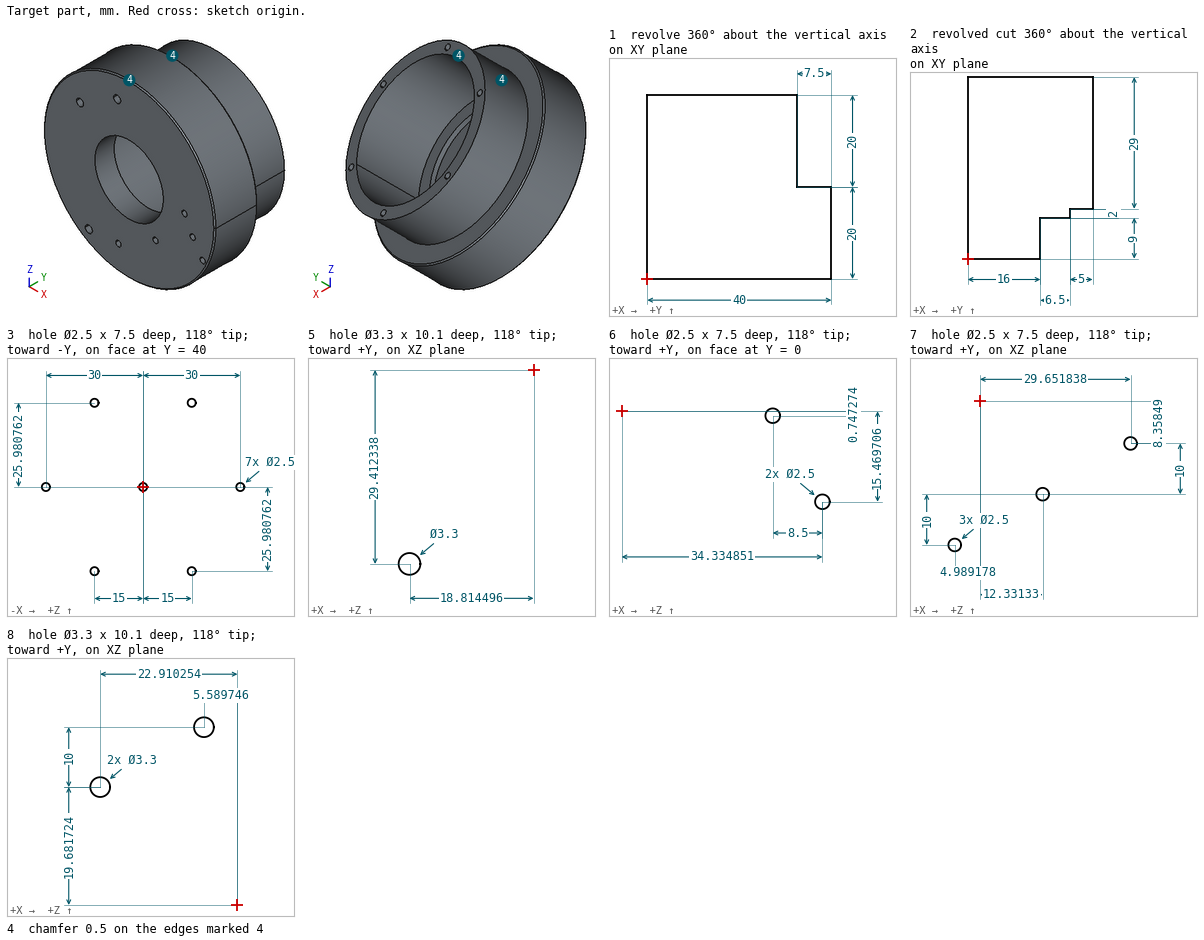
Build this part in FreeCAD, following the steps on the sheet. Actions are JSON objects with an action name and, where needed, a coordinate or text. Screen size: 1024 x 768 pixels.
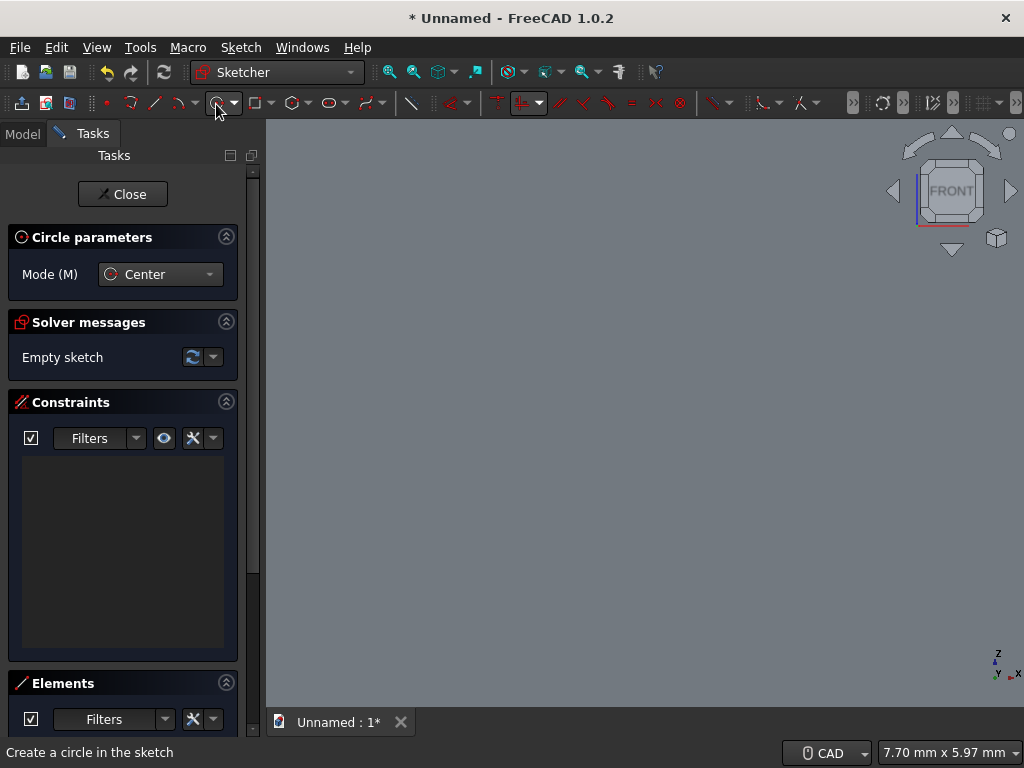
{"action": "left_click", "coordinate": [576, 394]}
{"action": "mouse_move", "coordinate": [691, 279]}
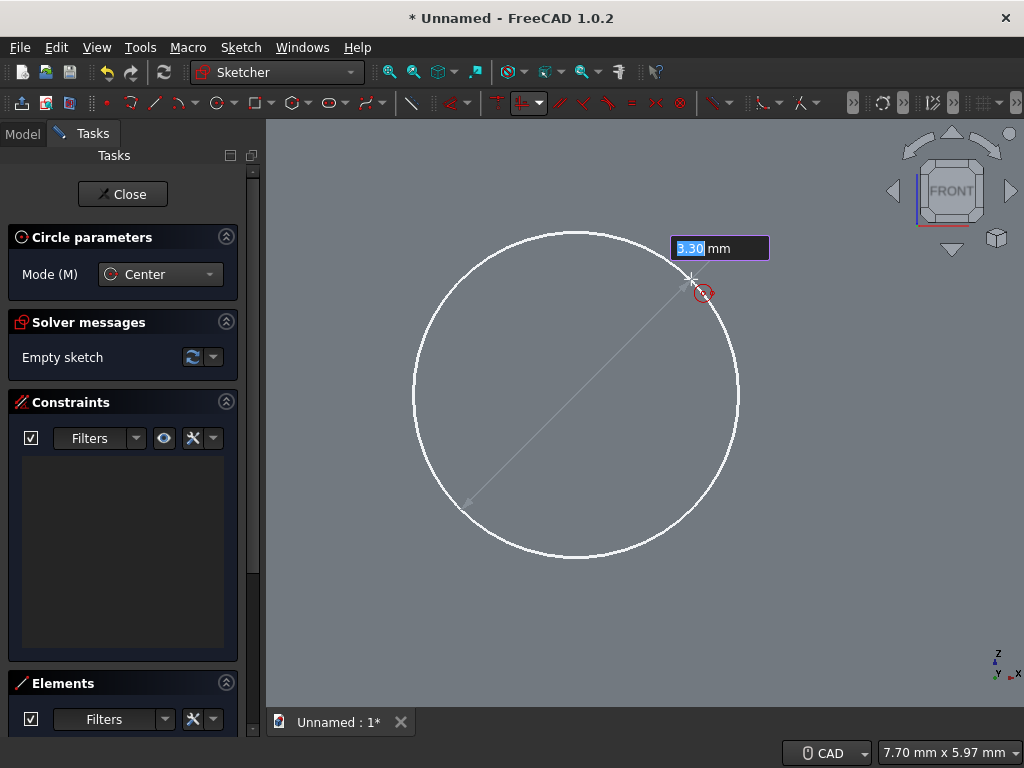
{"action": "type", "text": "3.3"}
{"action": "key", "text": "Return"}
{"action": "key", "text": "Escape"}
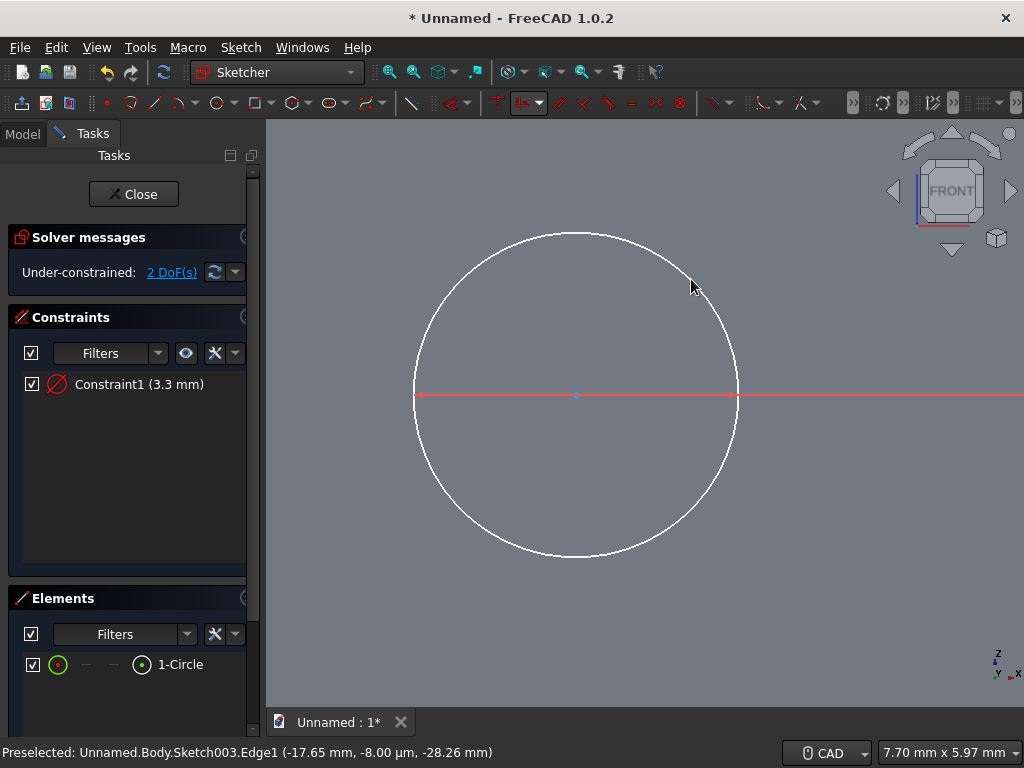
{"action": "left_click", "coordinate": [450, 104]}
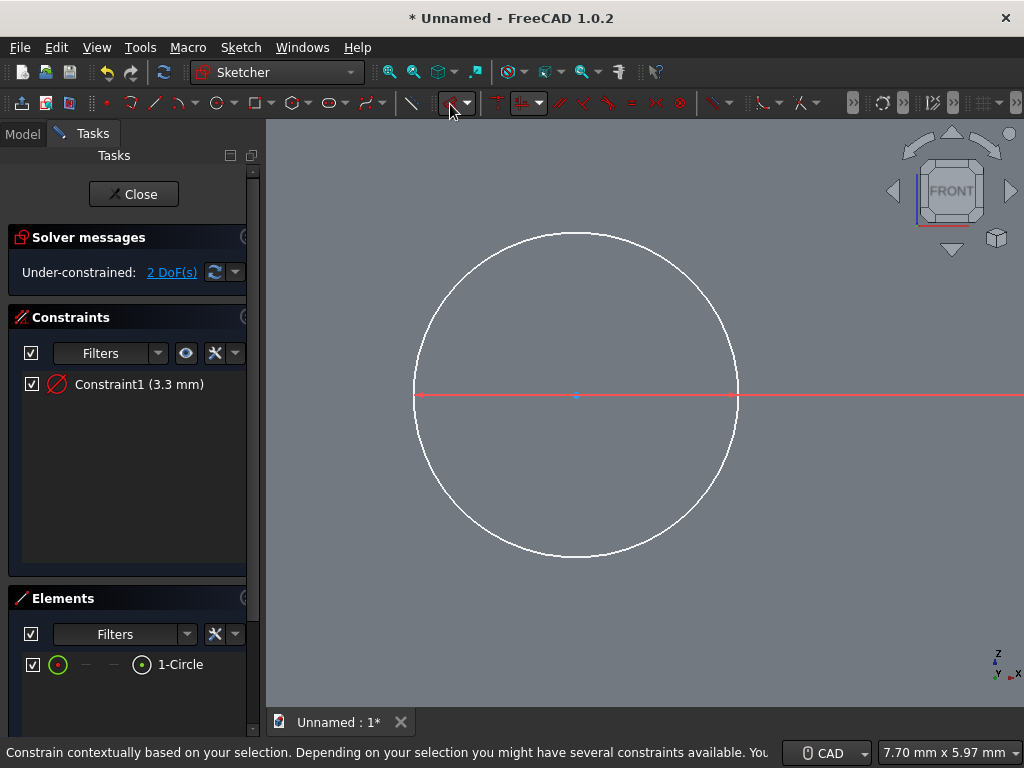
{"action": "left_click", "coordinate": [576, 395]}
{"action": "left_click", "coordinate": [717, 429]}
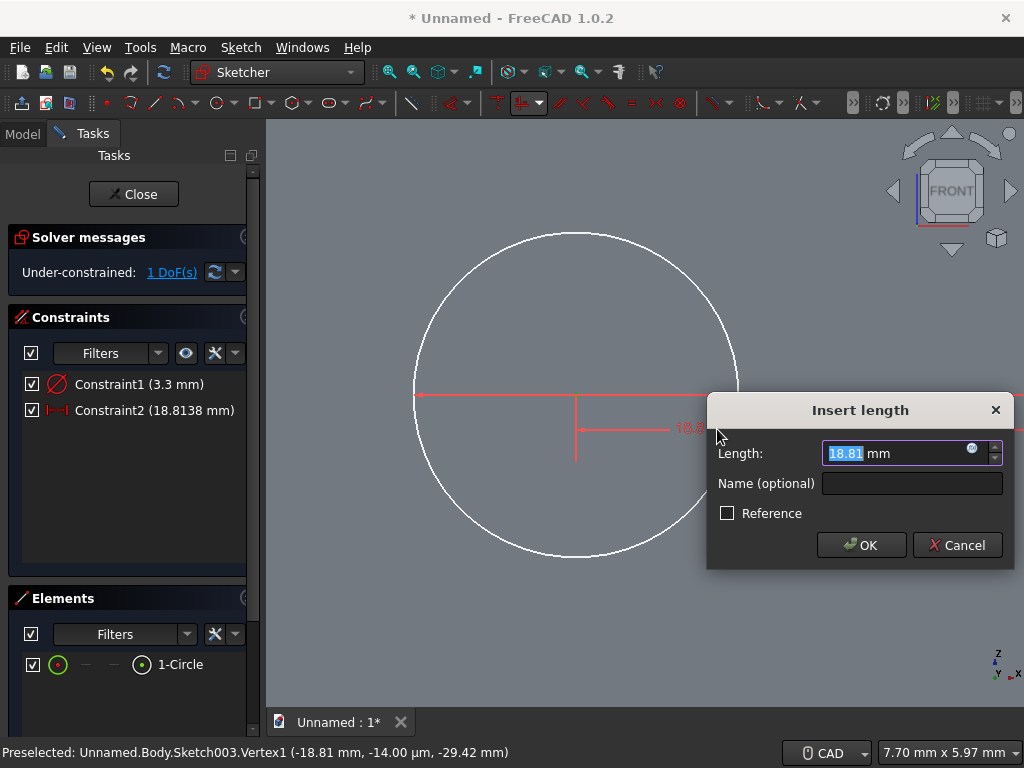
{"action": "type", "text": "18.814496"}
{"action": "key", "text": "Return"}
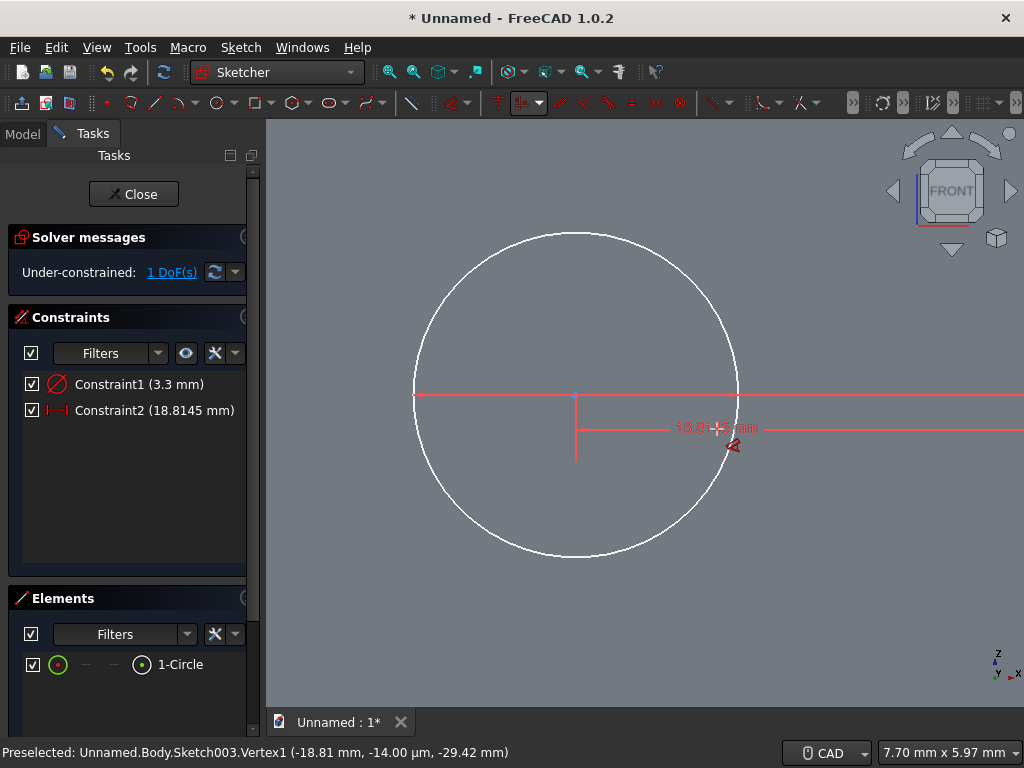
{"action": "left_click", "coordinate": [576, 395]}
{"action": "left_click", "coordinate": [542, 271]}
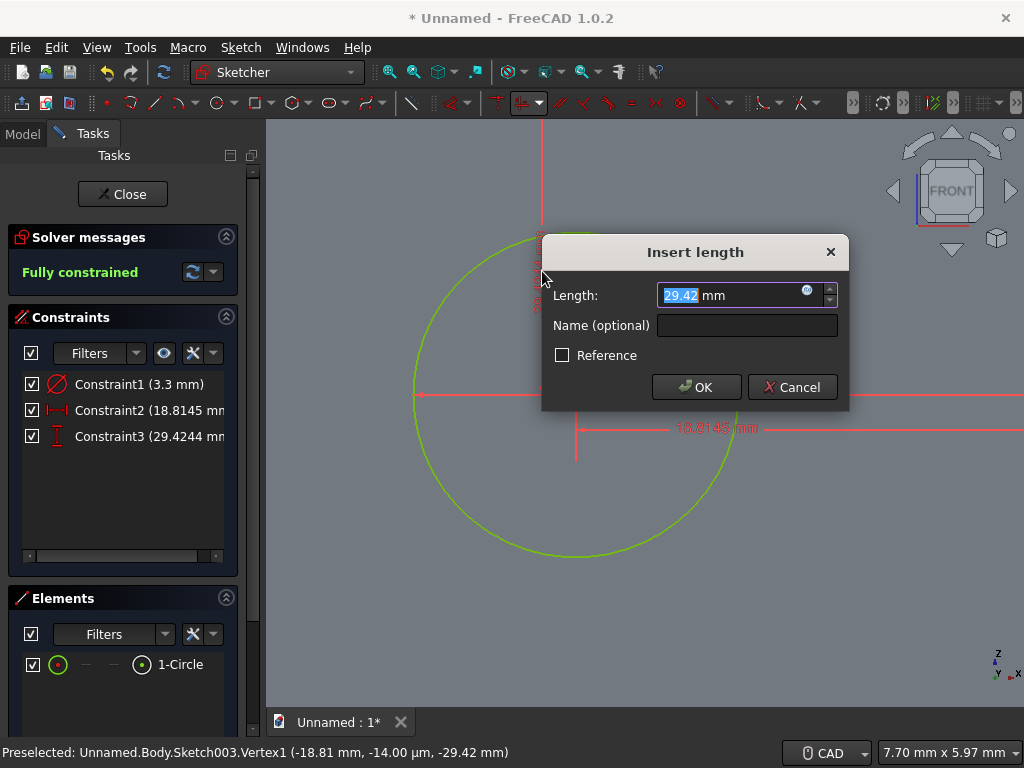
{"action": "type", "text": "29.412338"}
{"action": "key", "text": "Return"}
{"action": "key", "text": "Escape"}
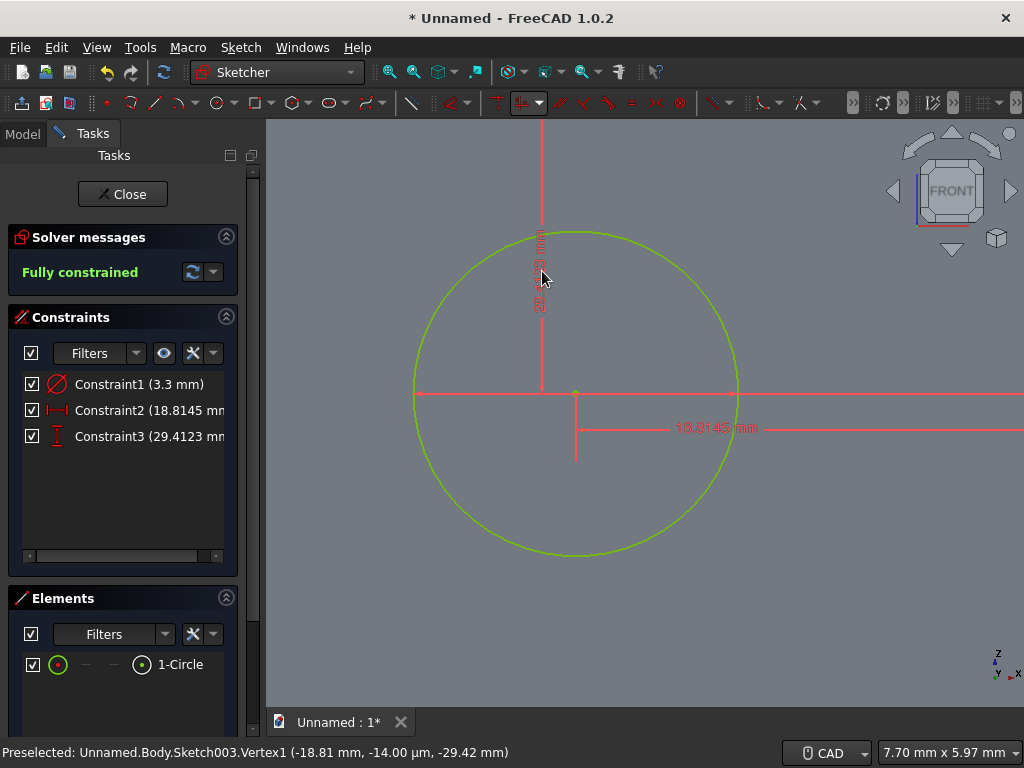
{"action": "left_click", "coordinate": [123, 194]}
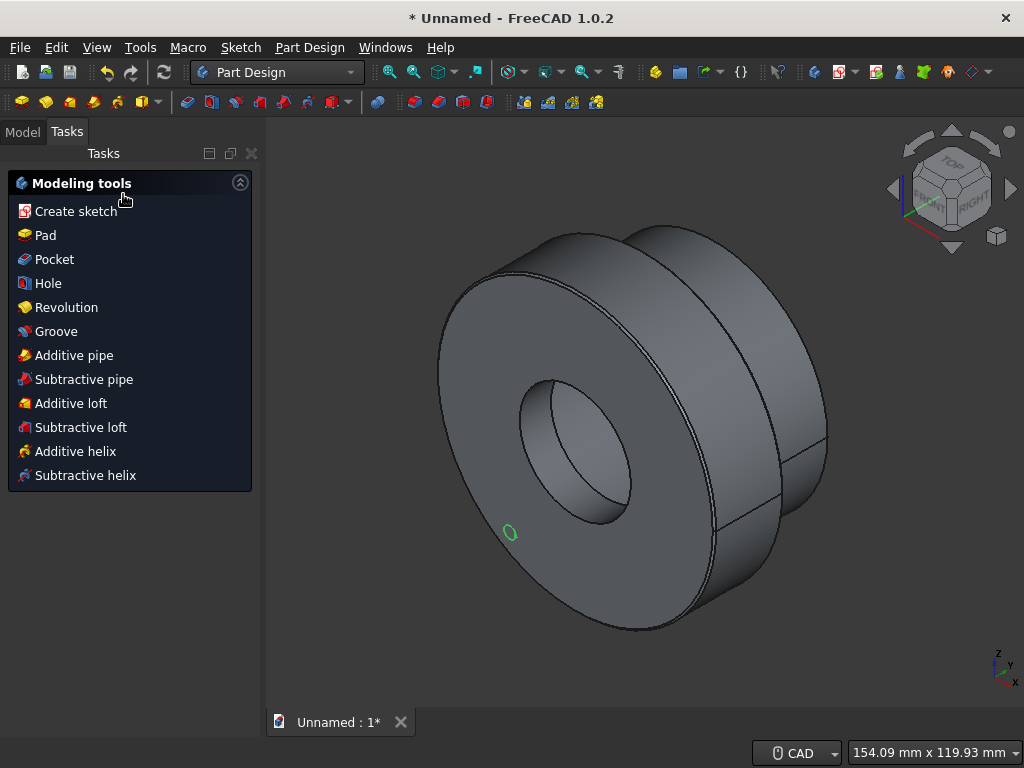
{"action": "left_click", "coordinate": [212, 102]}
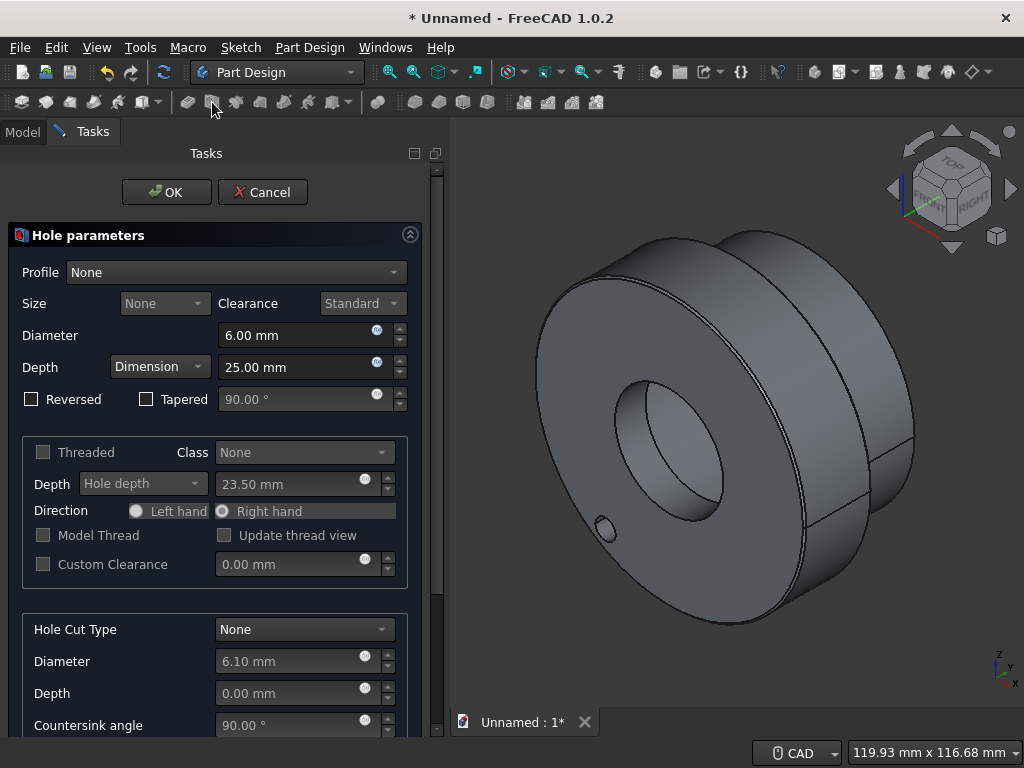
{"action": "triple_click", "coordinate": [305, 335]}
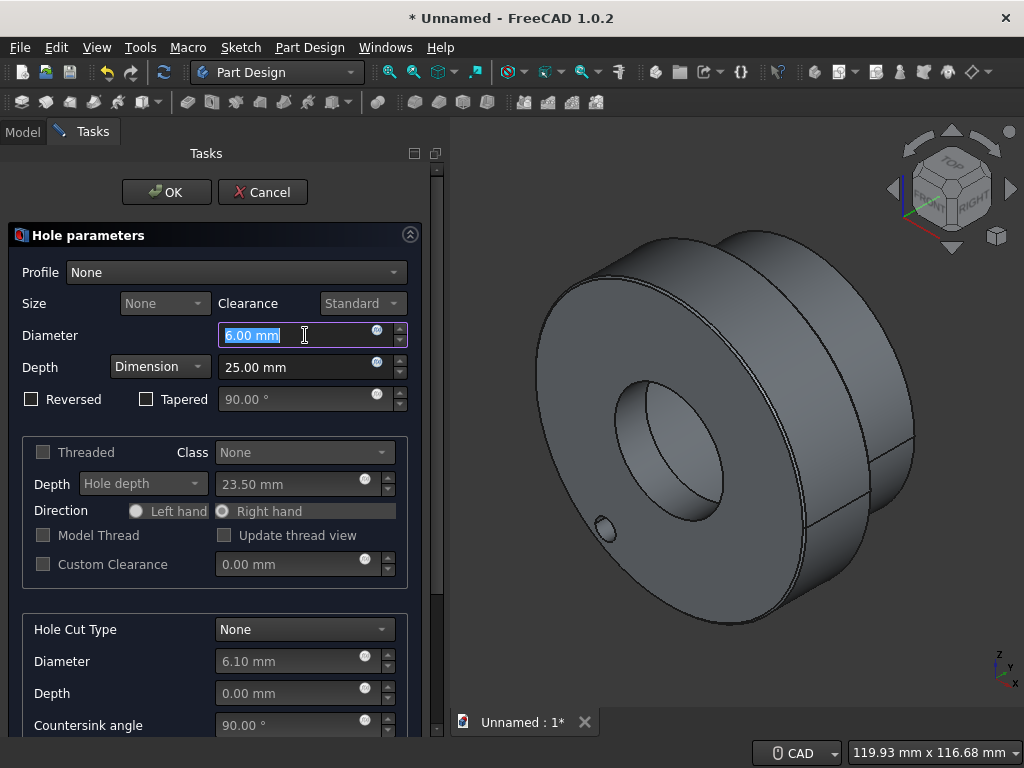
{"action": "type", "text": "3.3"}
{"action": "key", "text": "Tab"}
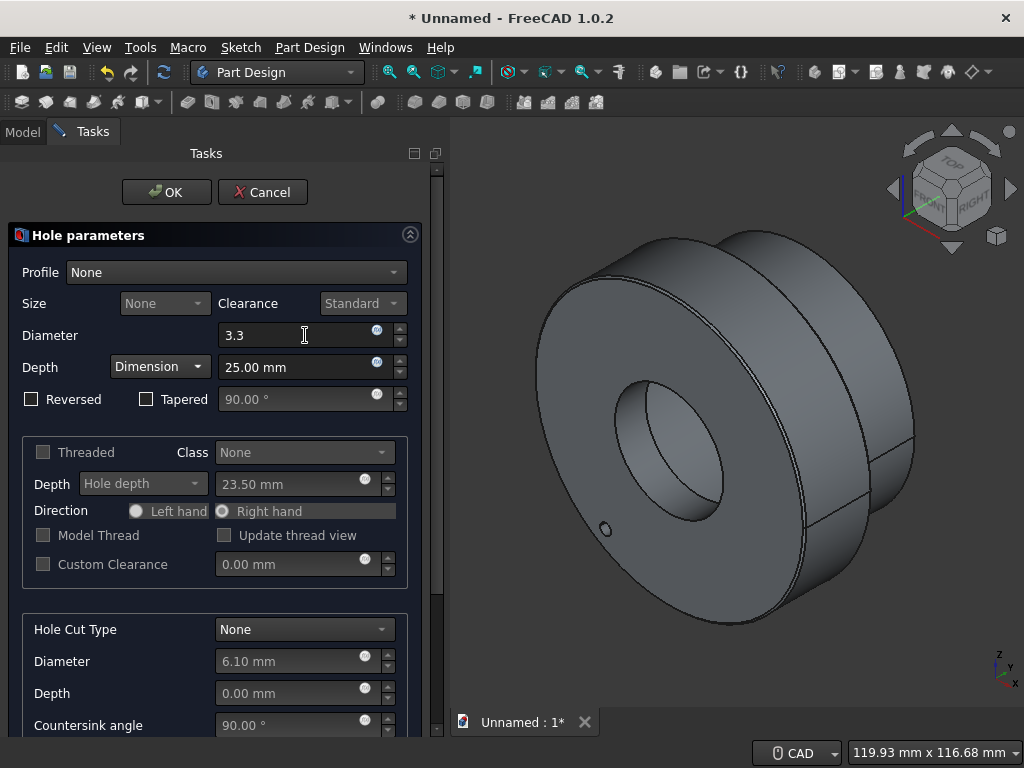
{"action": "triple_click", "coordinate": [305, 367]}